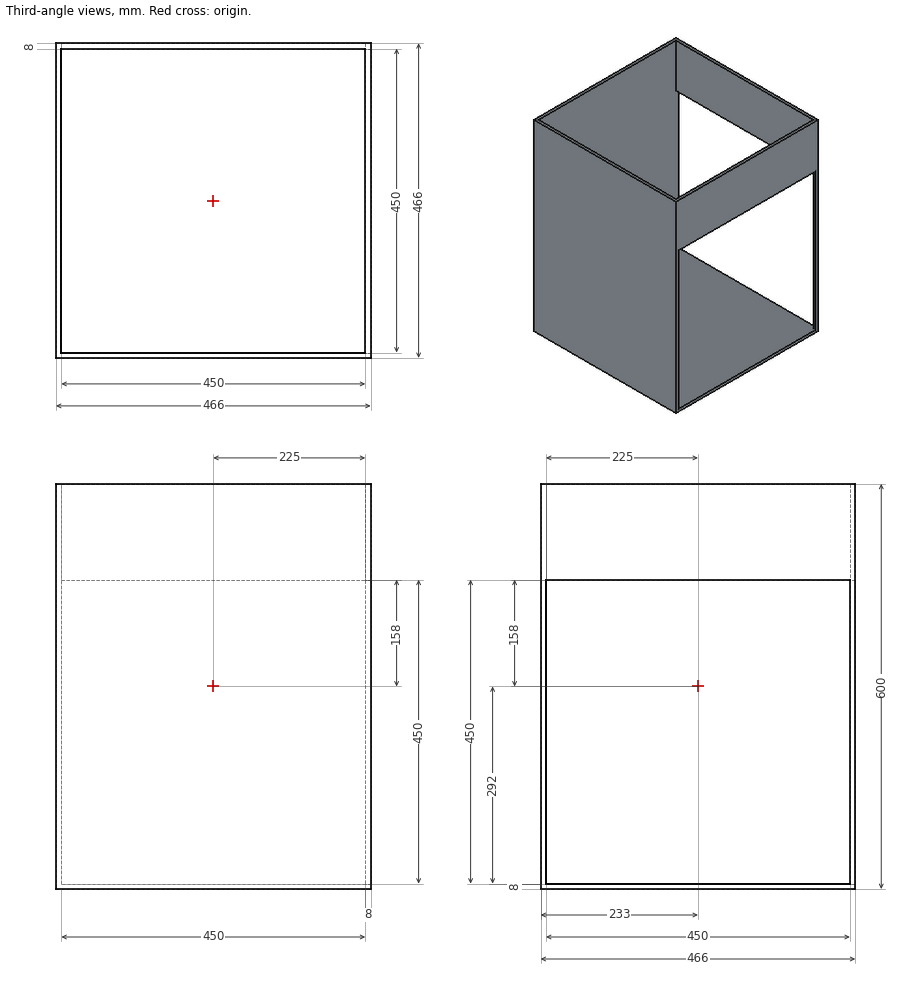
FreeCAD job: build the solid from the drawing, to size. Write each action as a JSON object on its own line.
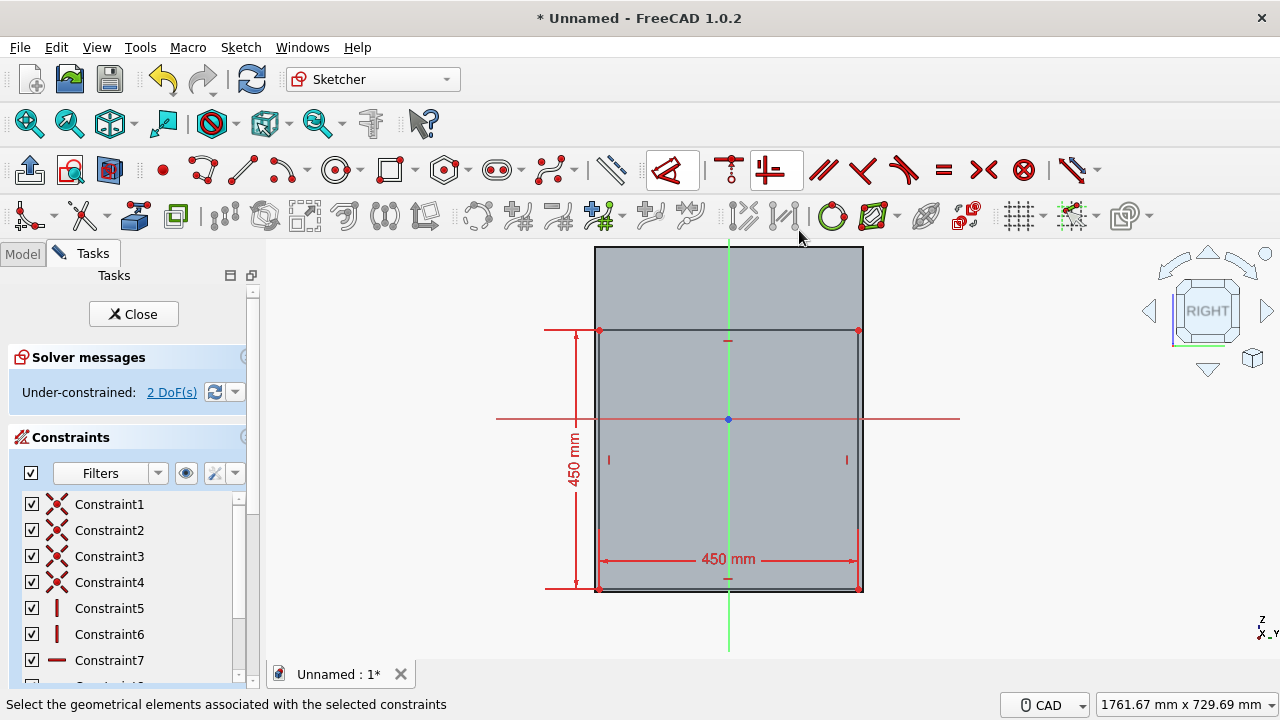
{"action": "left_click", "coordinate": [599, 330]}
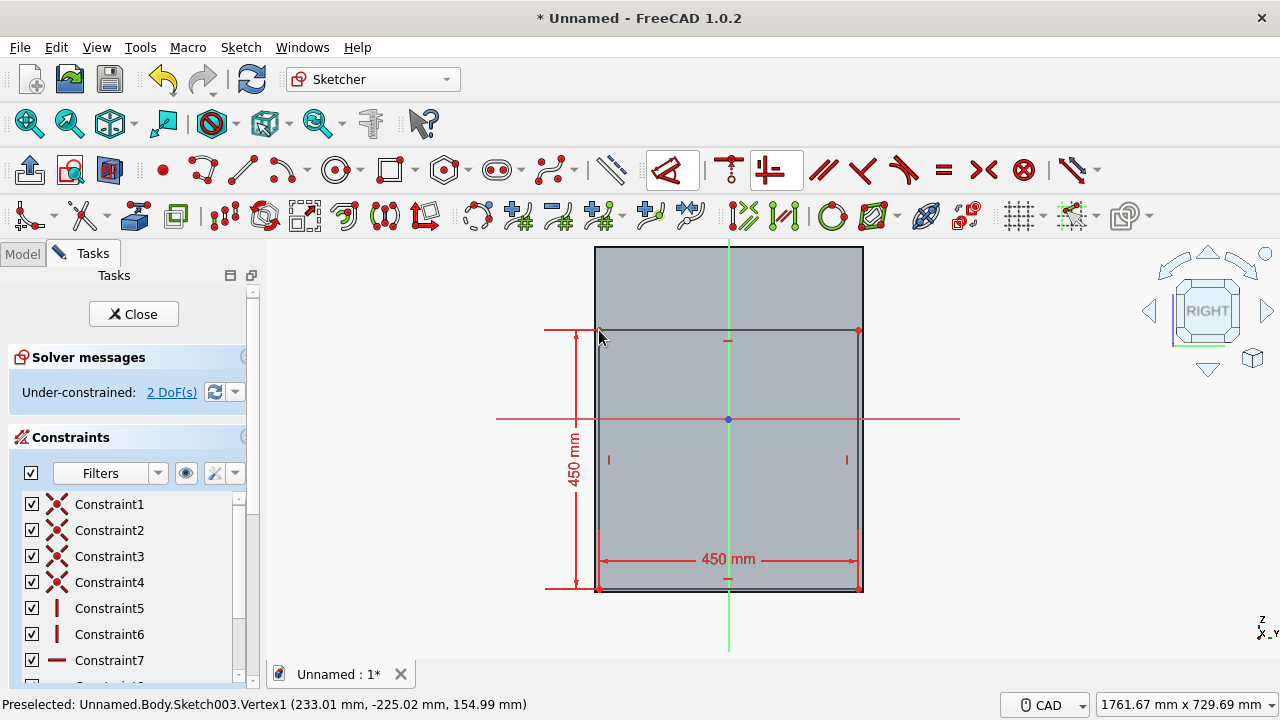
{"action": "left_click", "coordinate": [694, 170]}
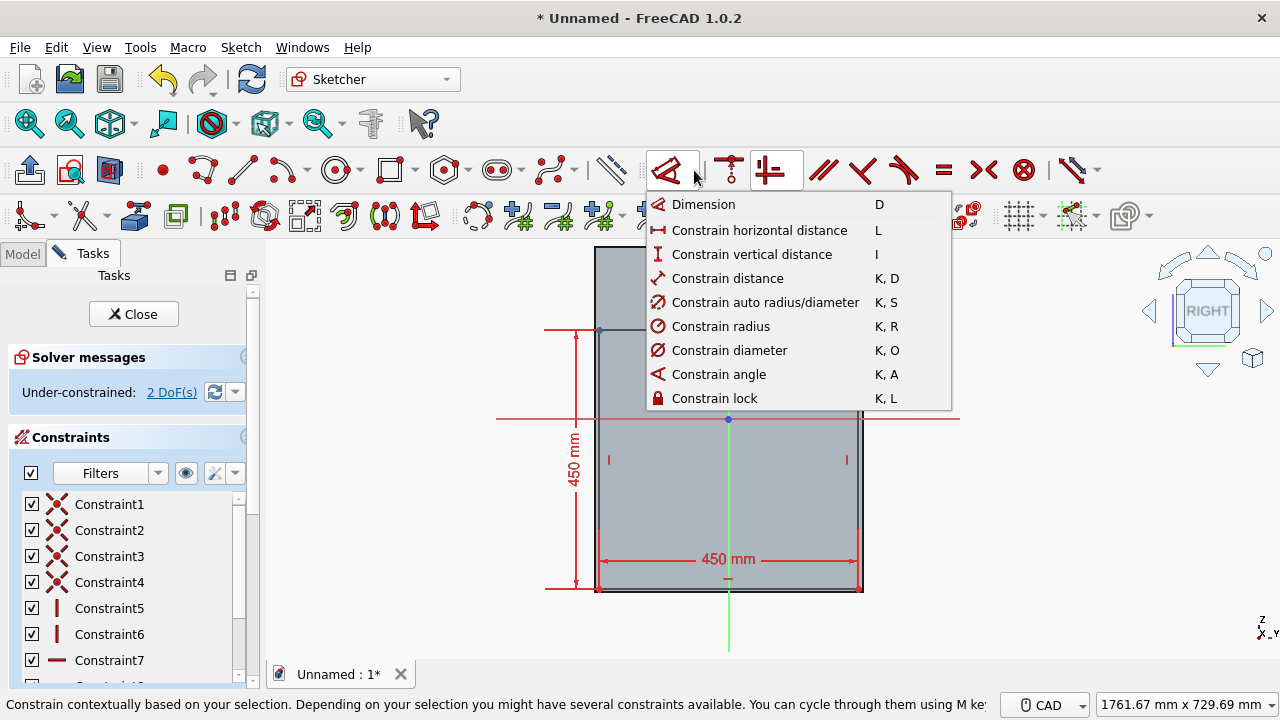
{"action": "left_click", "coordinate": [799, 230]}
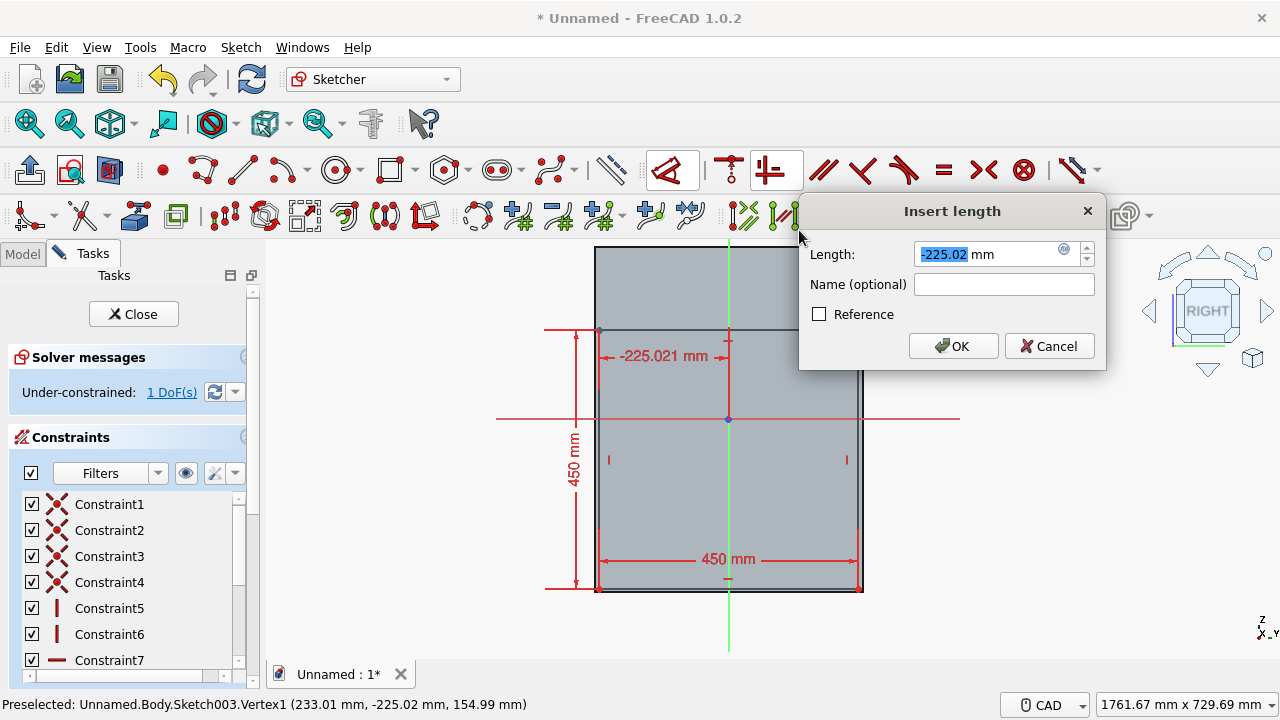
{"action": "type", "text": "-225"}
{"action": "key", "text": "Return"}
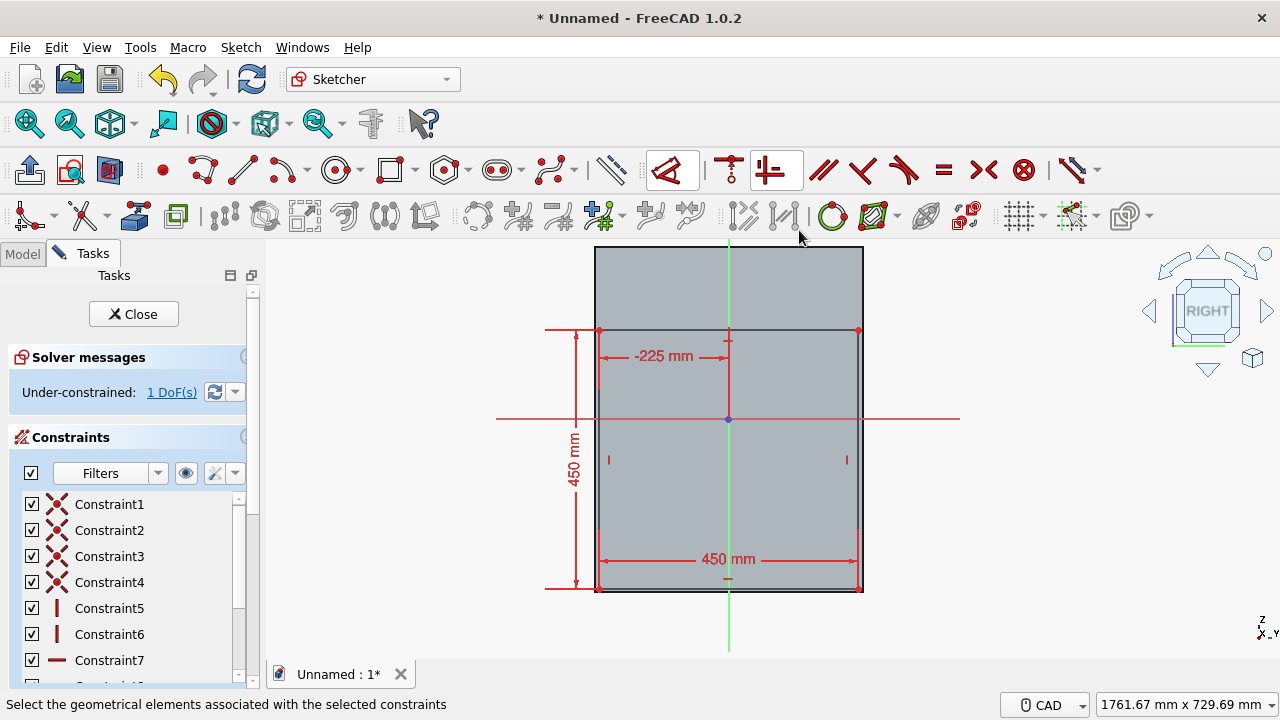
{"action": "left_click", "coordinate": [599, 330]}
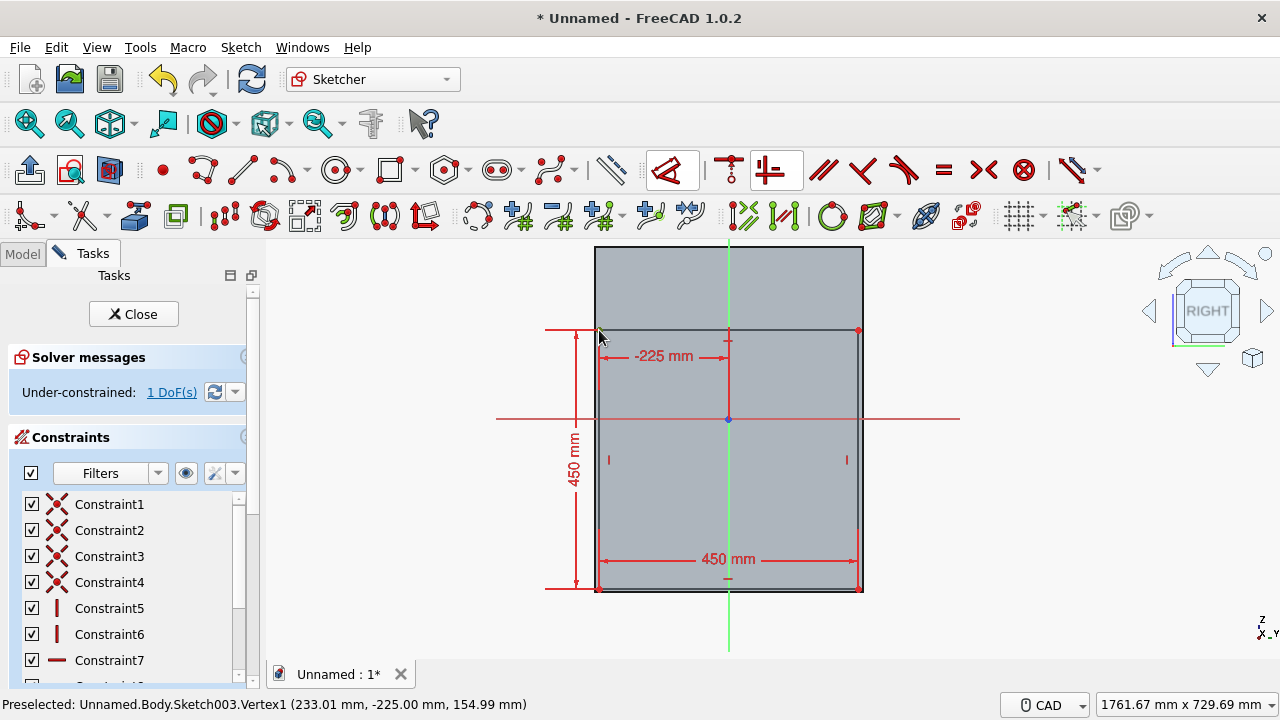
{"action": "left_click", "coordinate": [694, 170]}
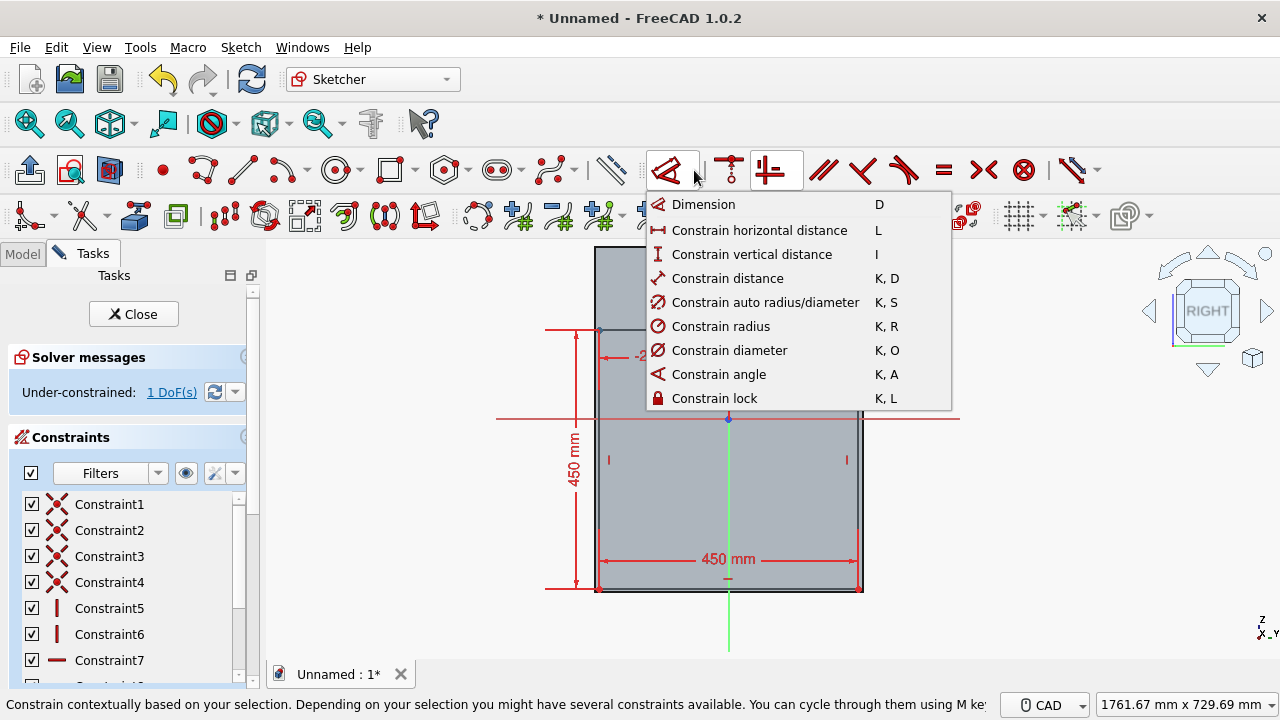
{"action": "left_click", "coordinate": [799, 254]}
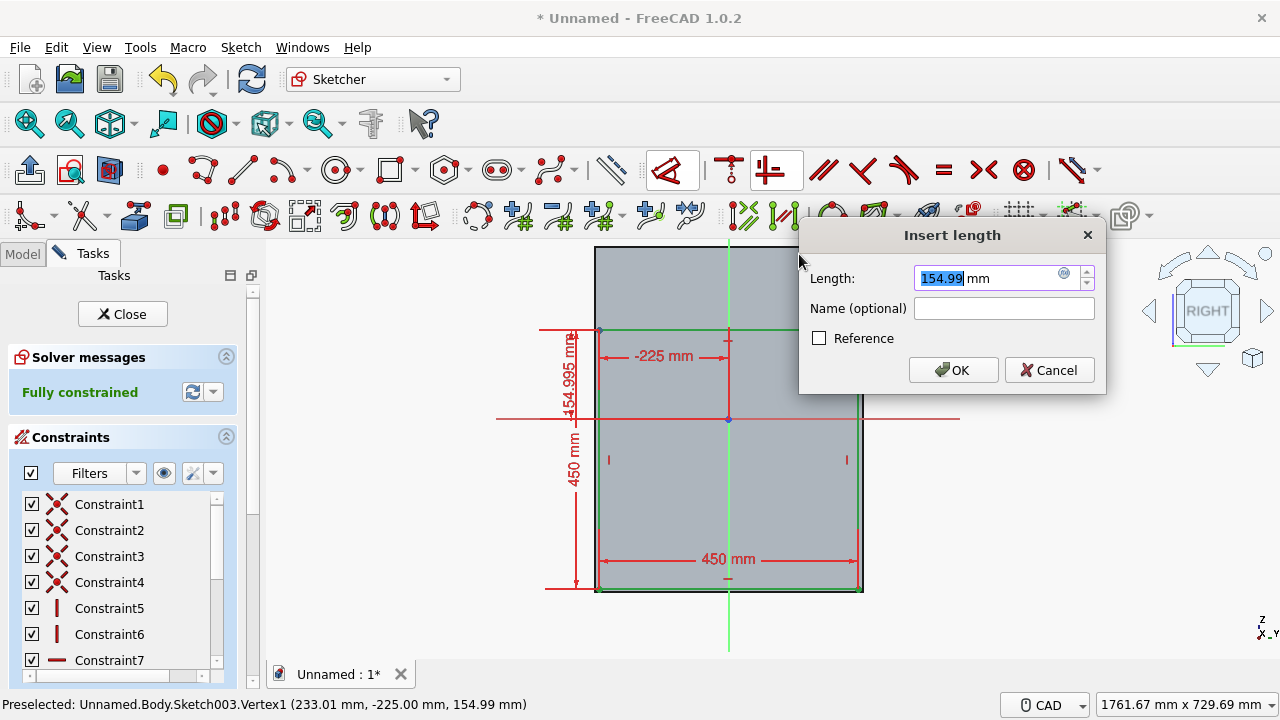
{"action": "type", "text": "158"}
{"action": "key", "text": "Return"}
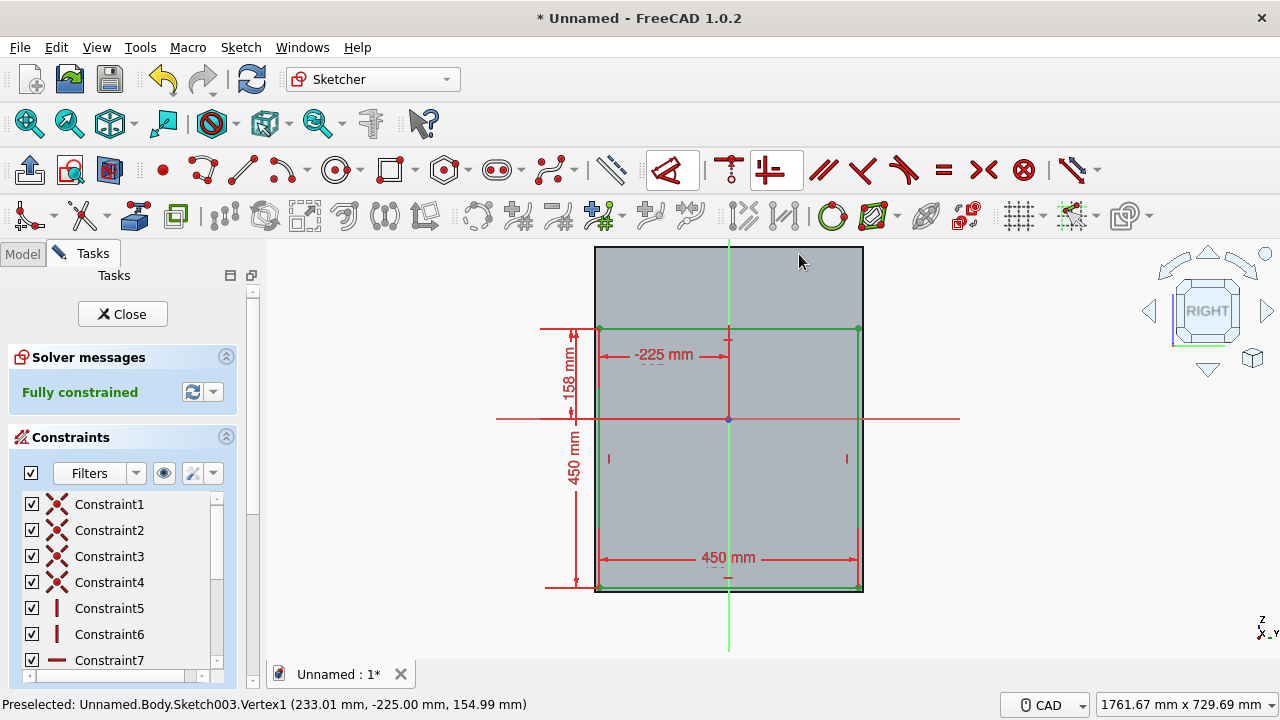
{"action": "left_click", "coordinate": [123, 314]}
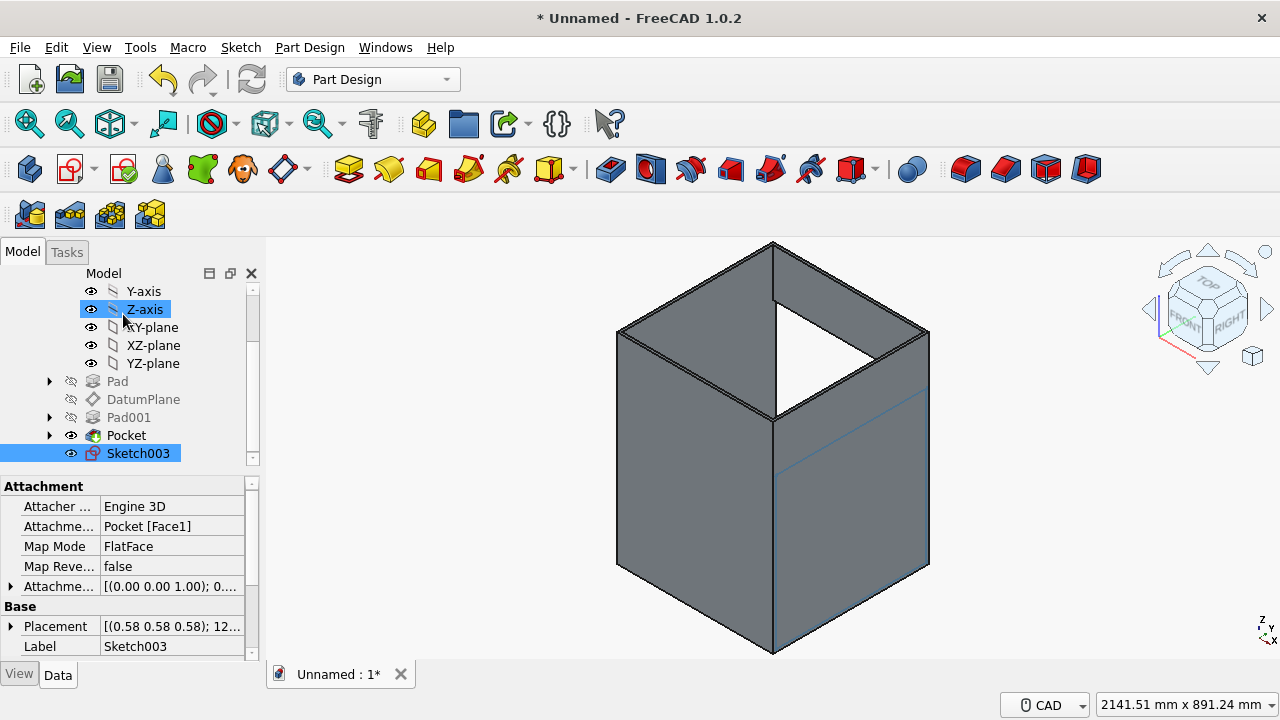
{"action": "left_click", "coordinate": [612, 170]}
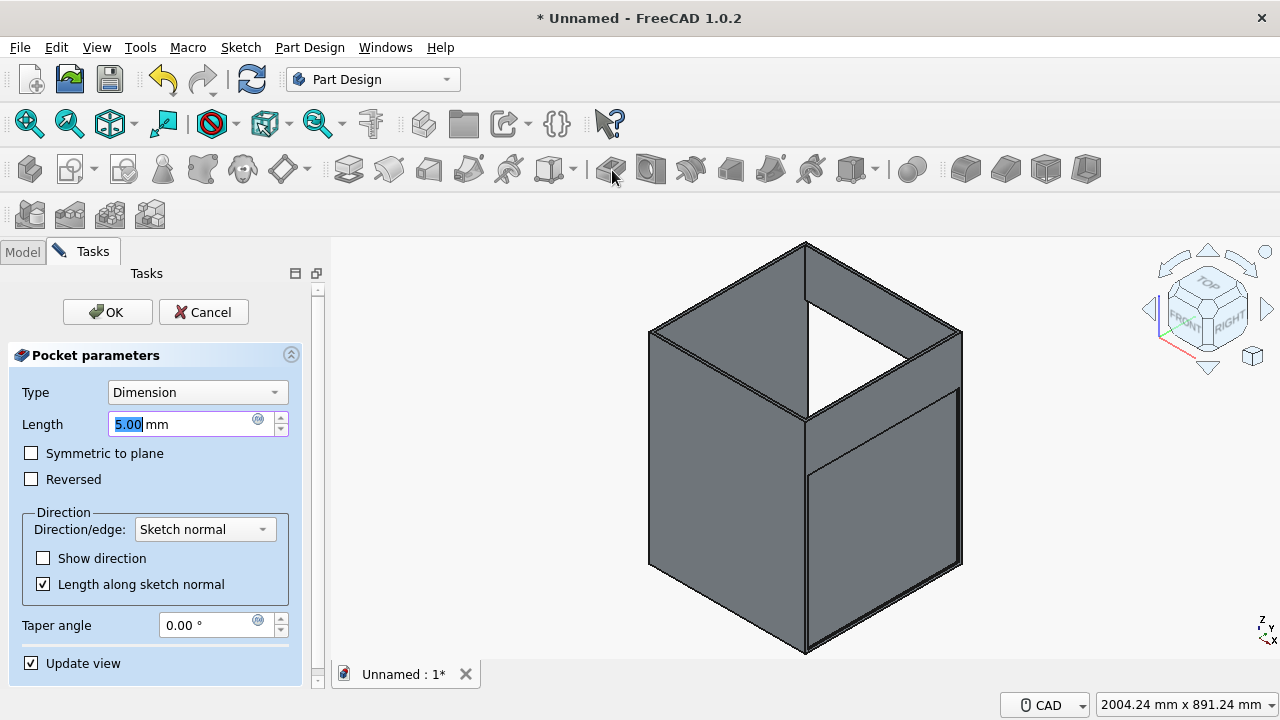
{"action": "type", "text": "8"}
{"action": "key", "text": "Tab"}